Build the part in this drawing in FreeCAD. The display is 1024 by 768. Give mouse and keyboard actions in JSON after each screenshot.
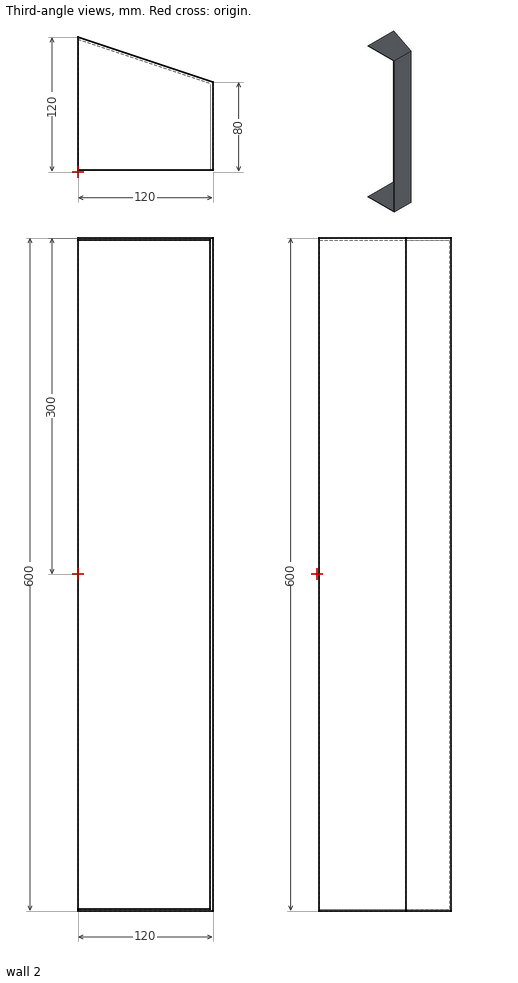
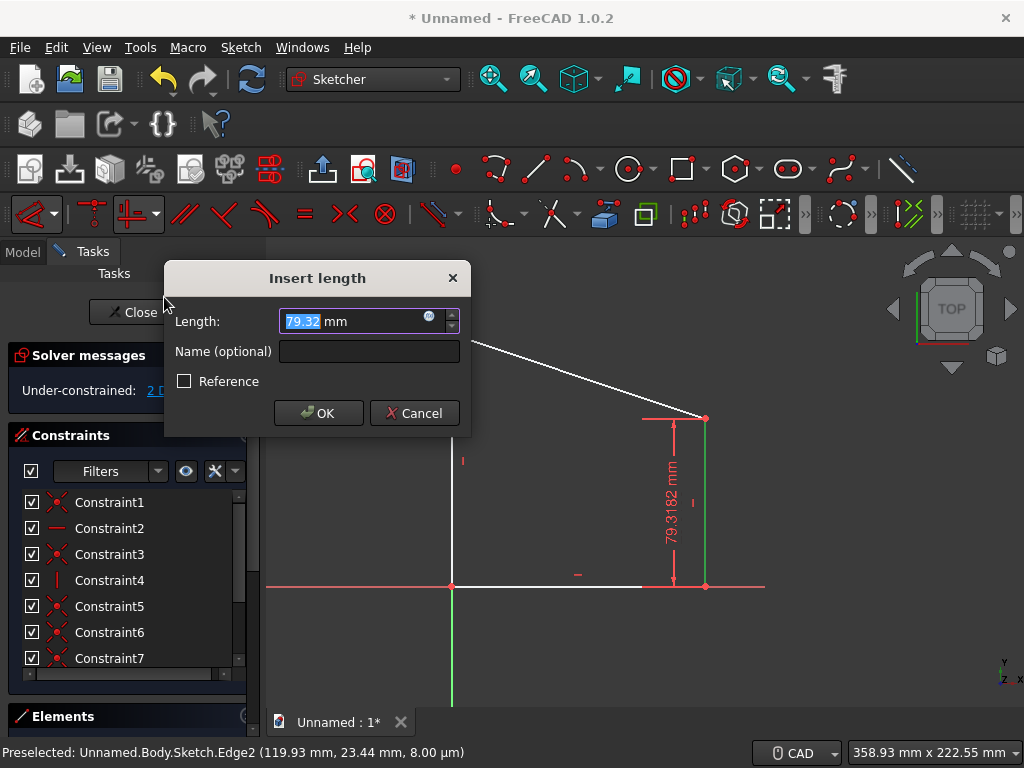
{"action": "type", "text": "80"}
{"action": "key", "text": "Return"}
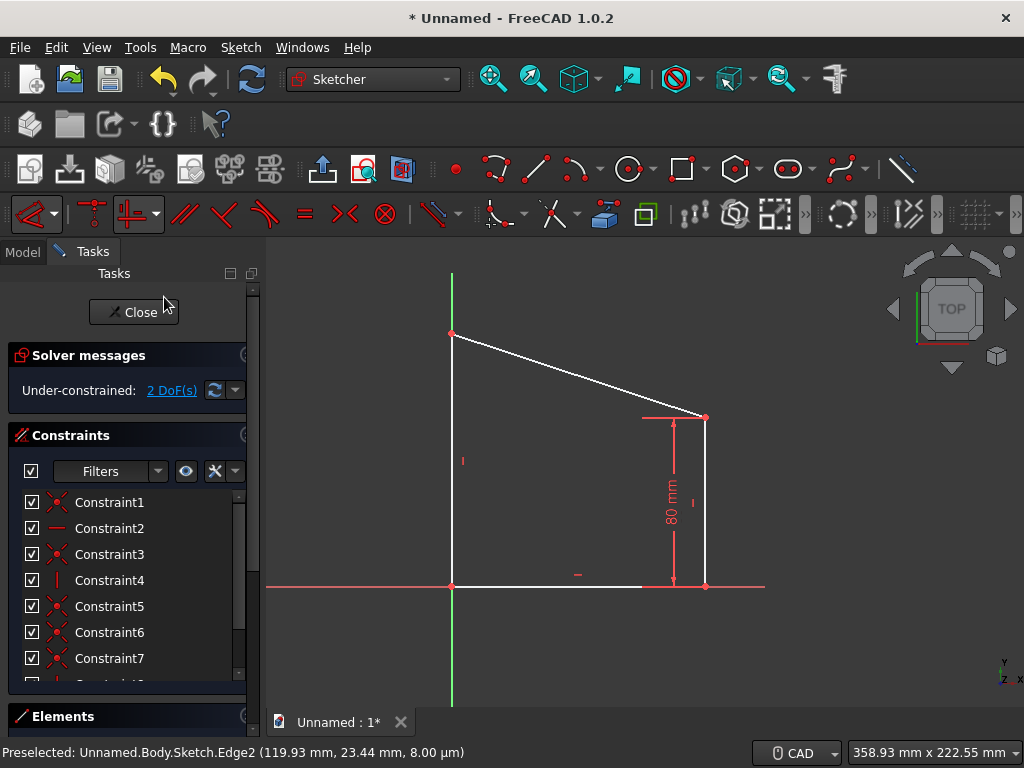
{"action": "left_click", "coordinate": [528, 587]}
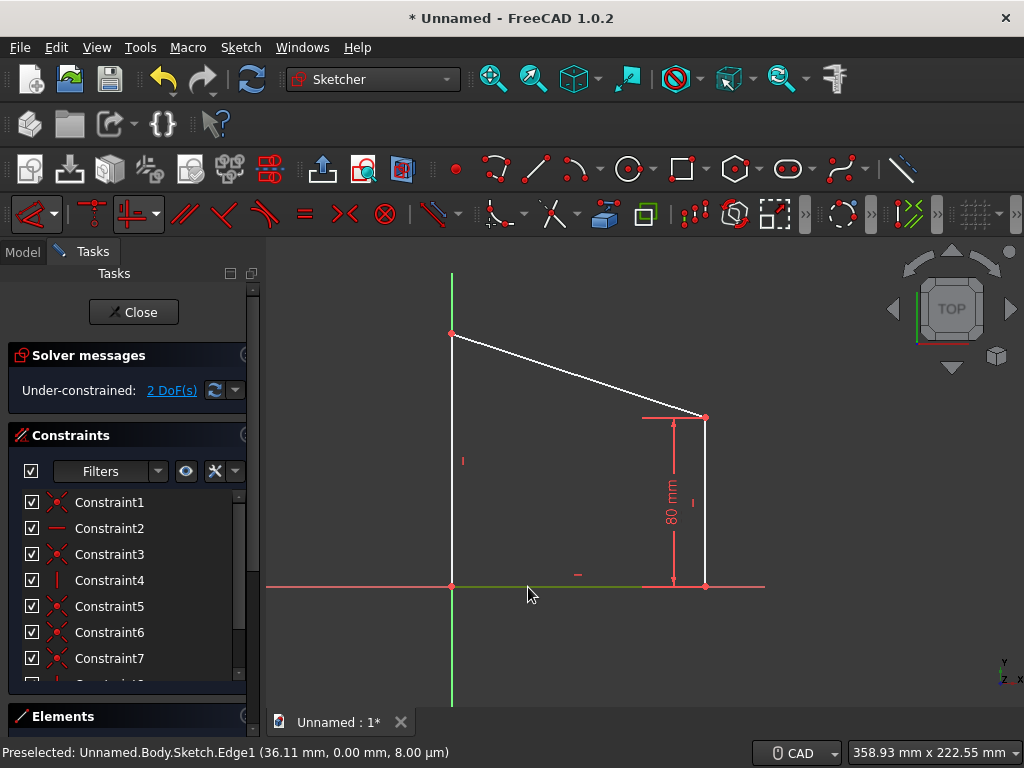
{"action": "left_click", "coordinate": [56, 214]}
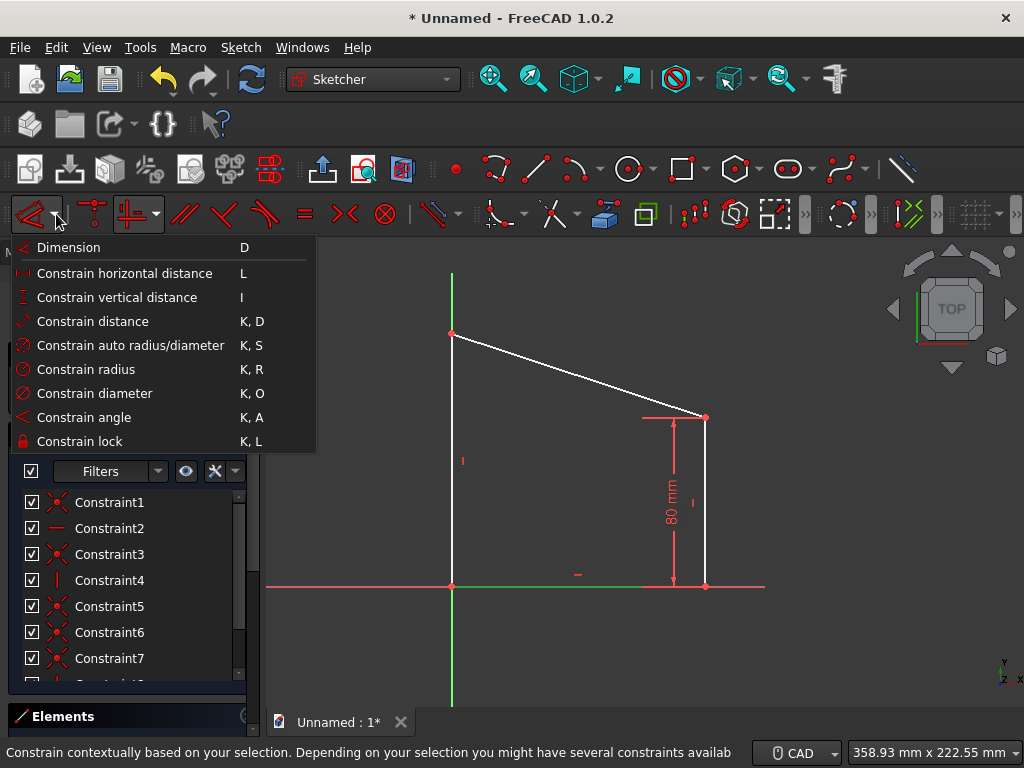
{"action": "left_click", "coordinate": [164, 273]}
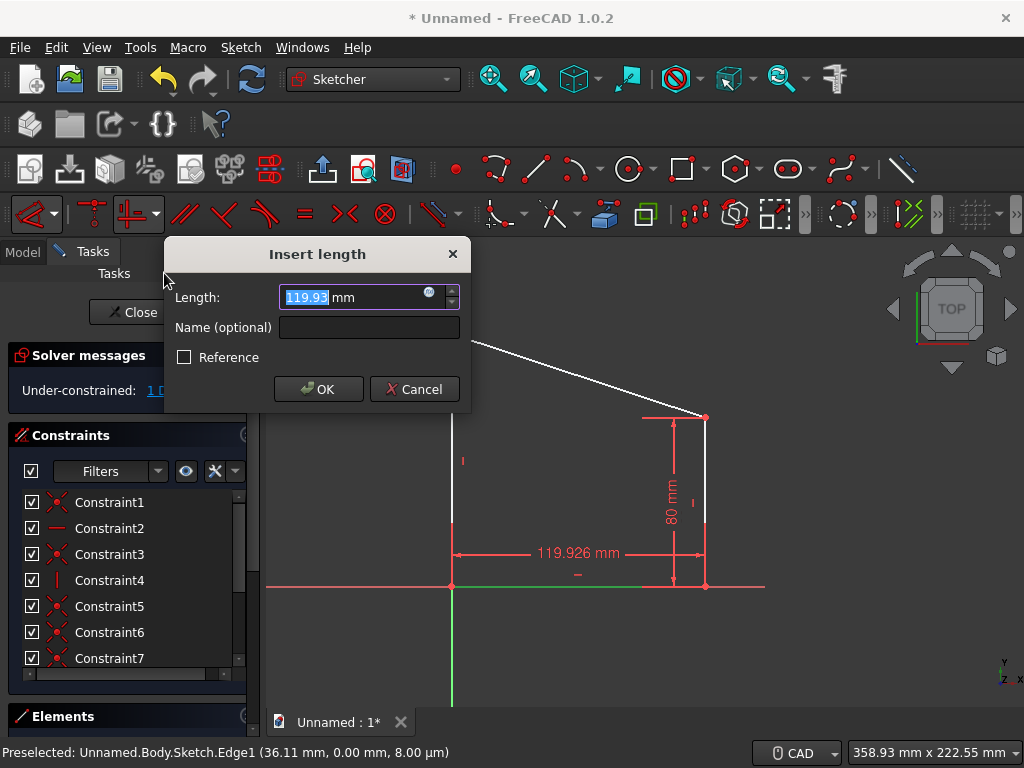
{"action": "type", "text": "120"}
{"action": "key", "text": "Return"}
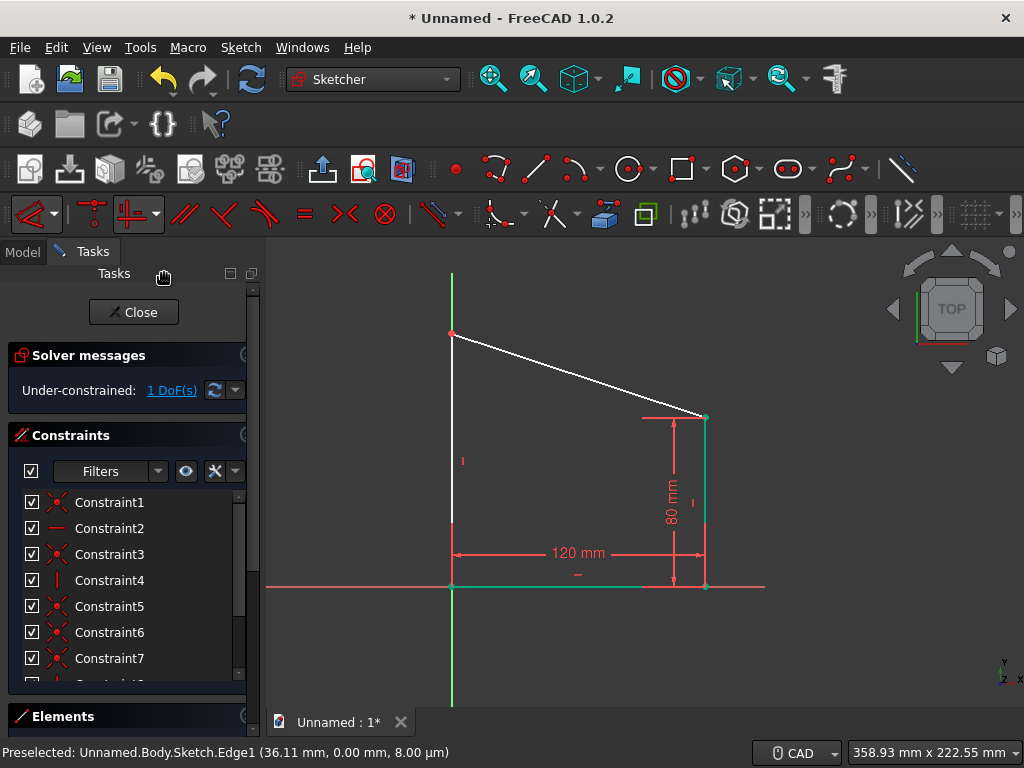
{"action": "left_click", "coordinate": [452, 410]}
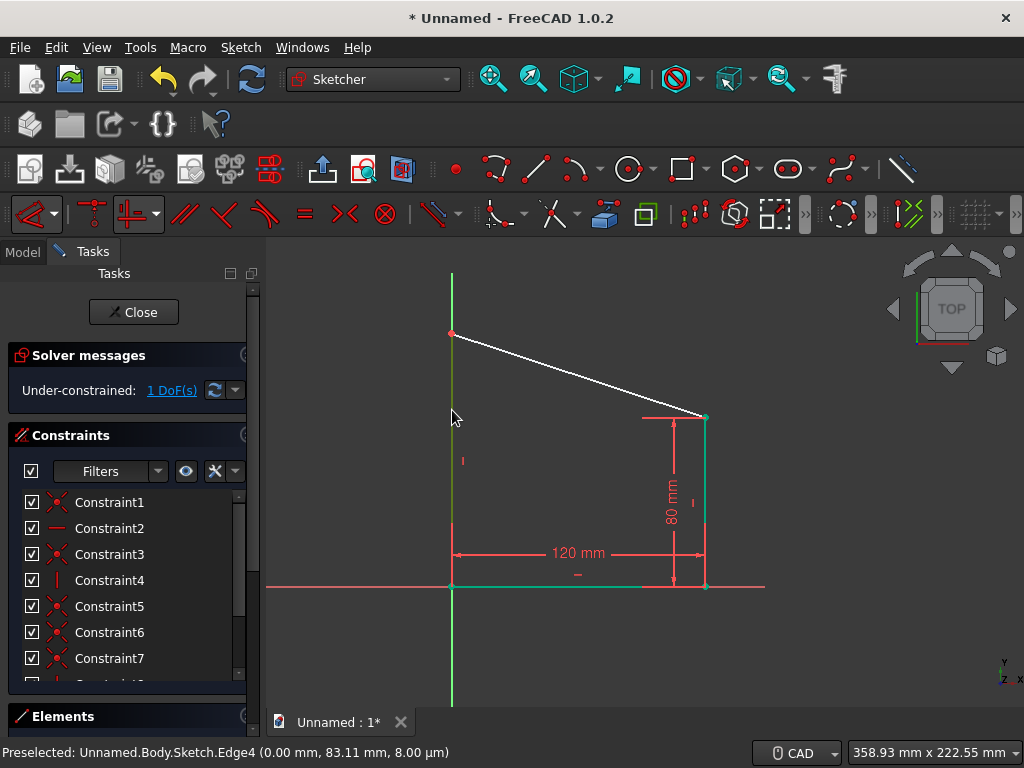
{"action": "left_click", "coordinate": [56, 214]}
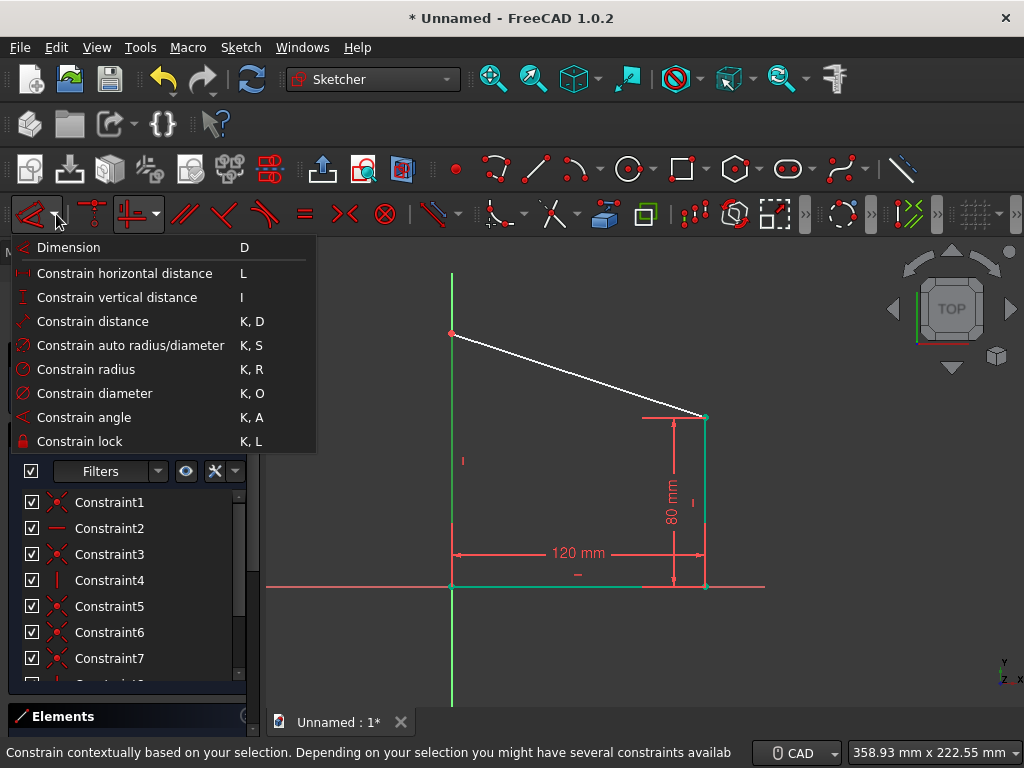
{"action": "left_click", "coordinate": [164, 297]}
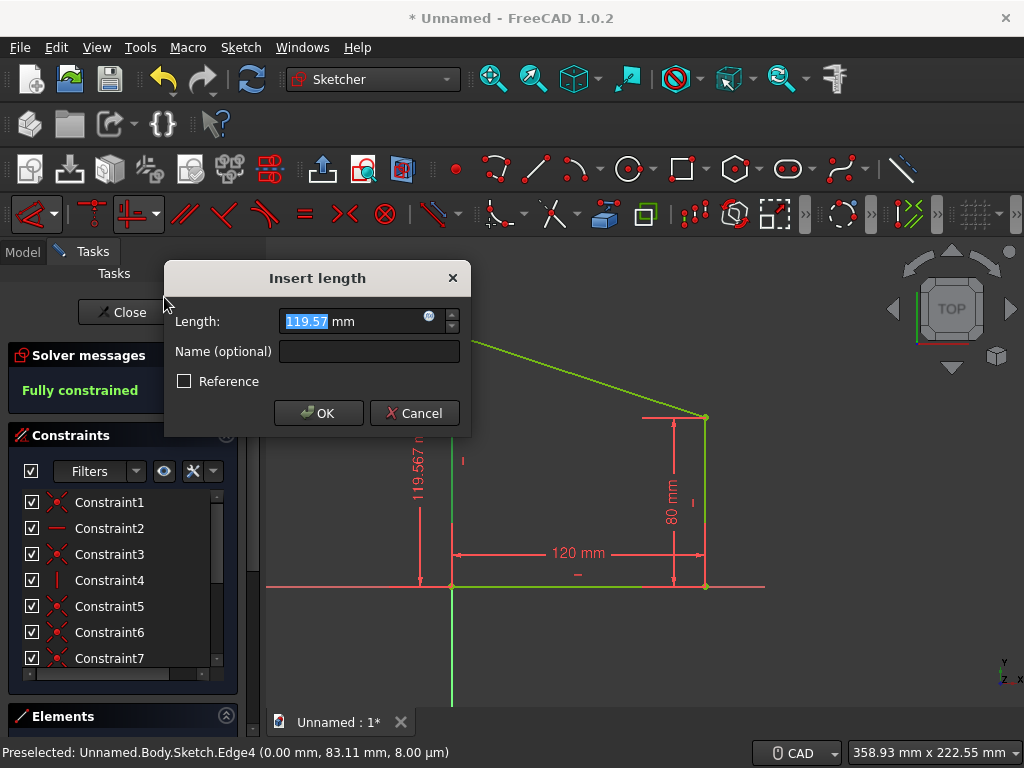
{"action": "type", "text": "120"}
{"action": "key", "text": "Return"}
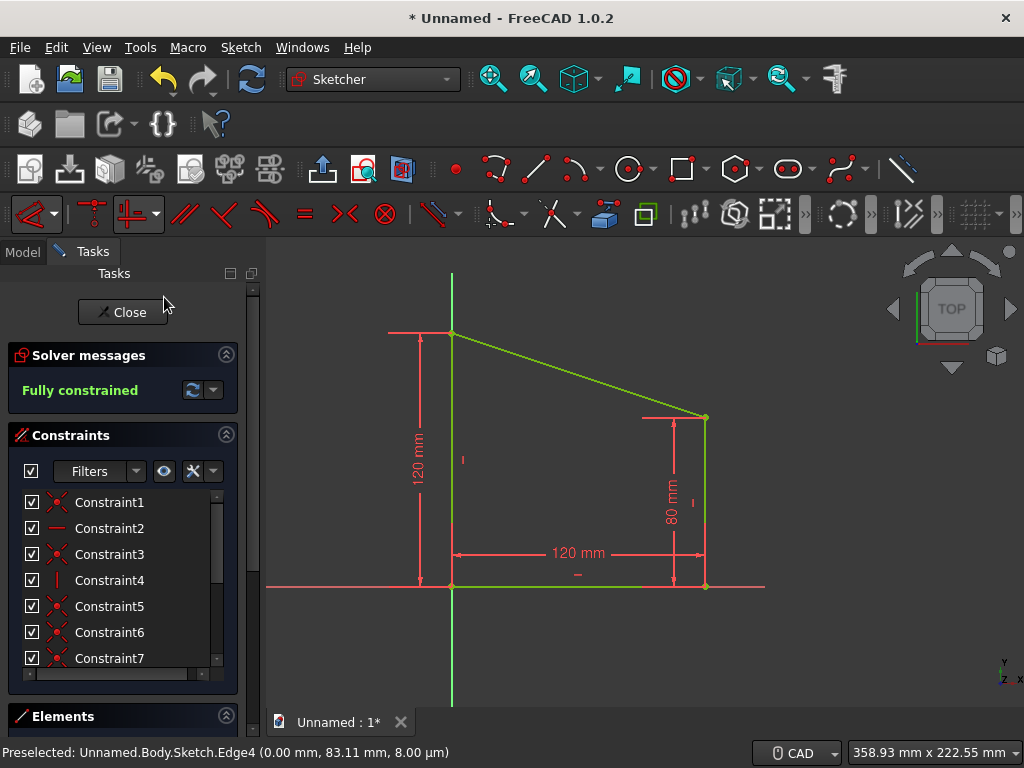
{"action": "left_click", "coordinate": [123, 312]}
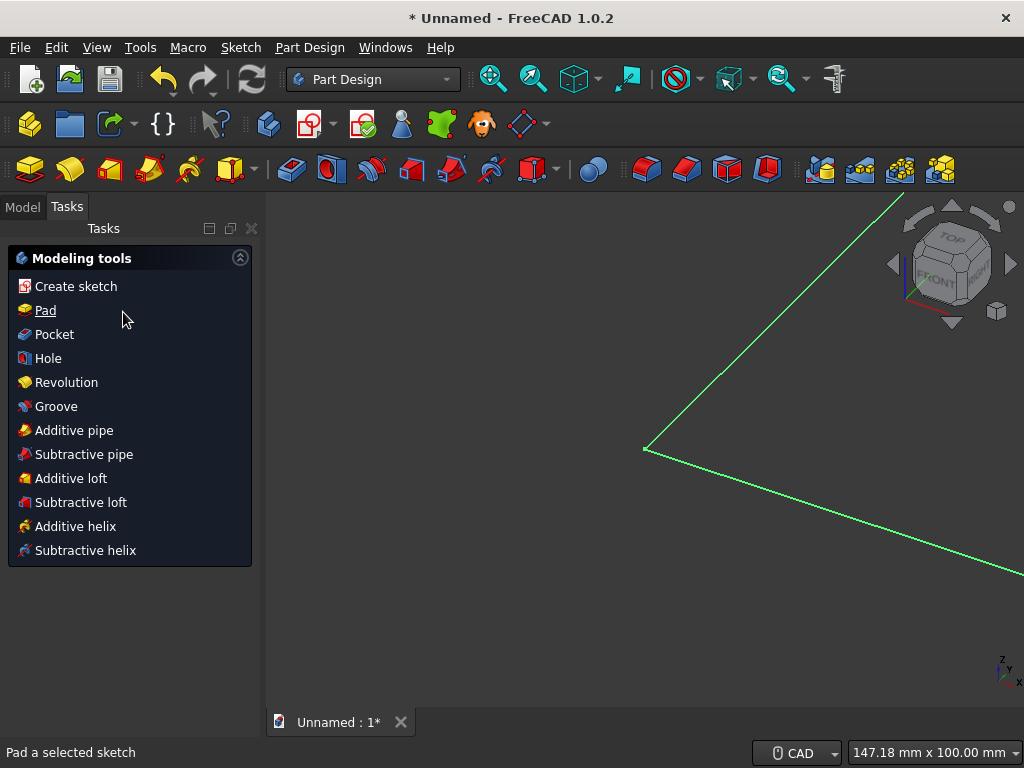
{"action": "left_click", "coordinate": [30, 170]}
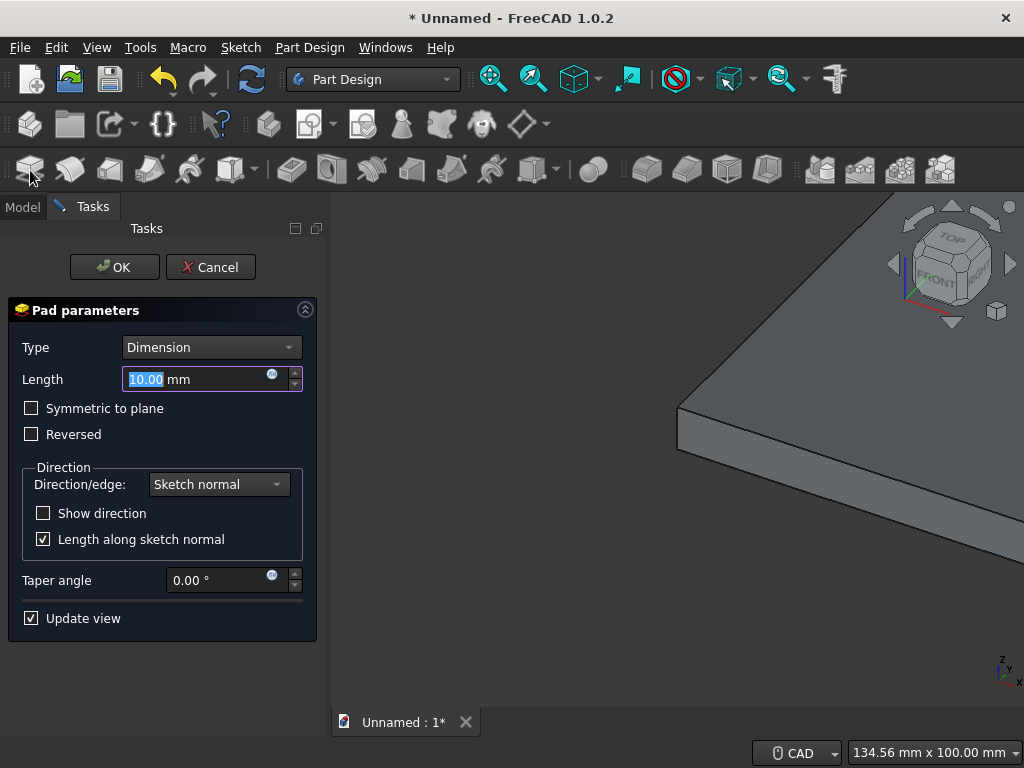
{"action": "type", "text": "600"}
{"action": "key", "text": "Tab"}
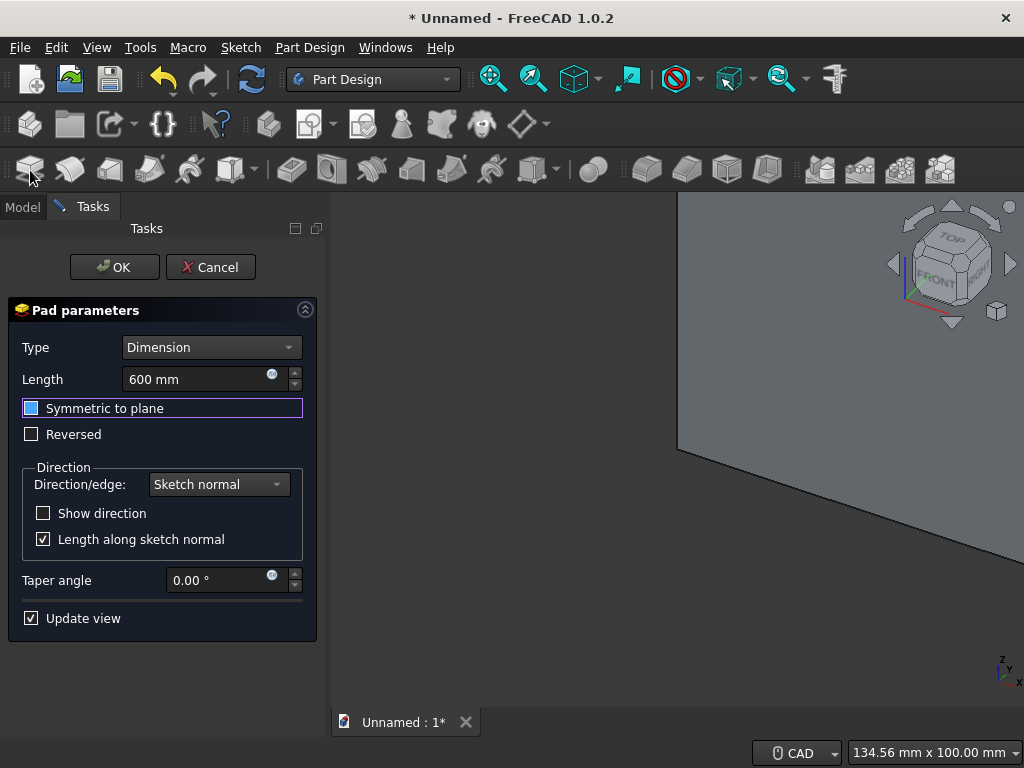
{"action": "left_click", "coordinate": [30, 408]}